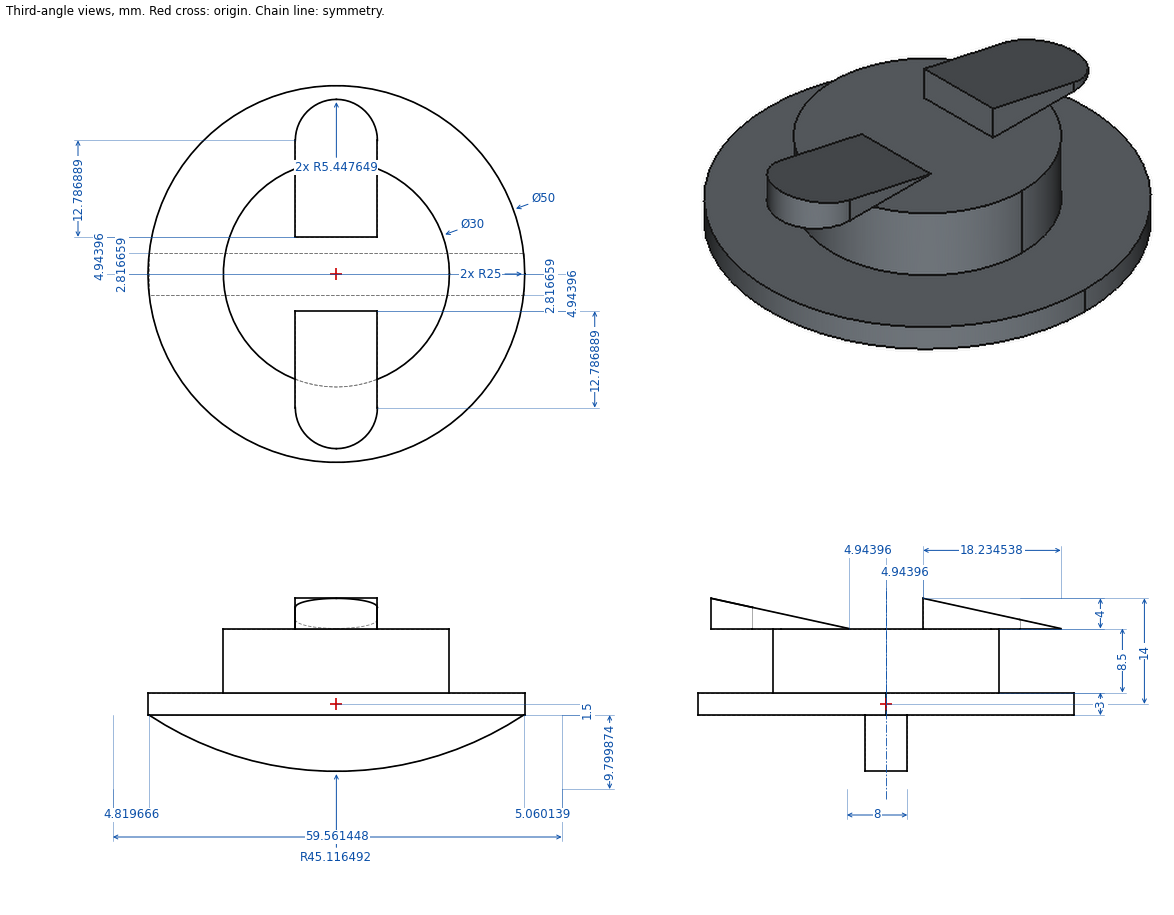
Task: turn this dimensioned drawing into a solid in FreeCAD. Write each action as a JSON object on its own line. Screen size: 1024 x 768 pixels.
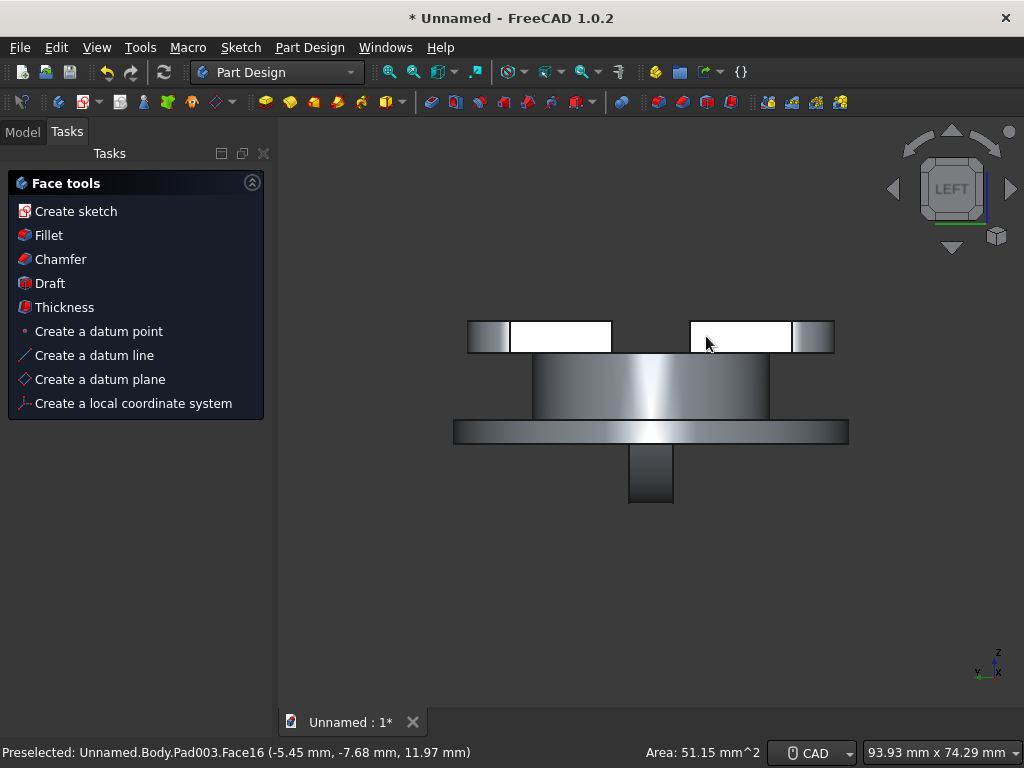
{"action": "left_click", "coordinate": [84, 102]}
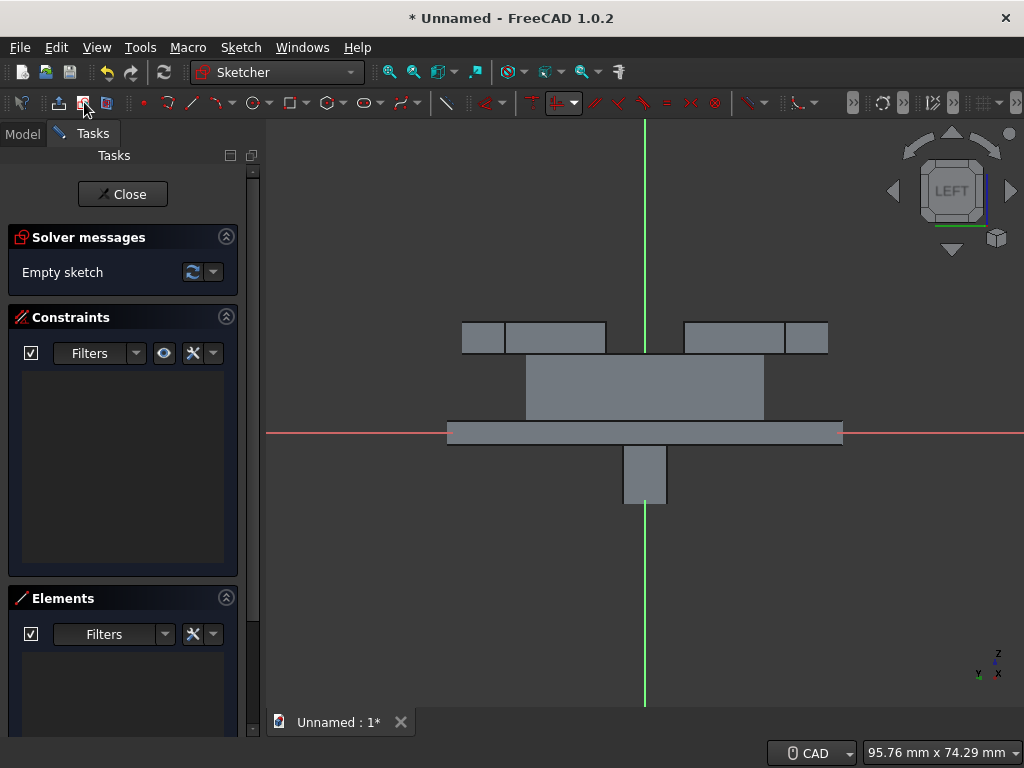
{"action": "left_click", "coordinate": [168, 104]}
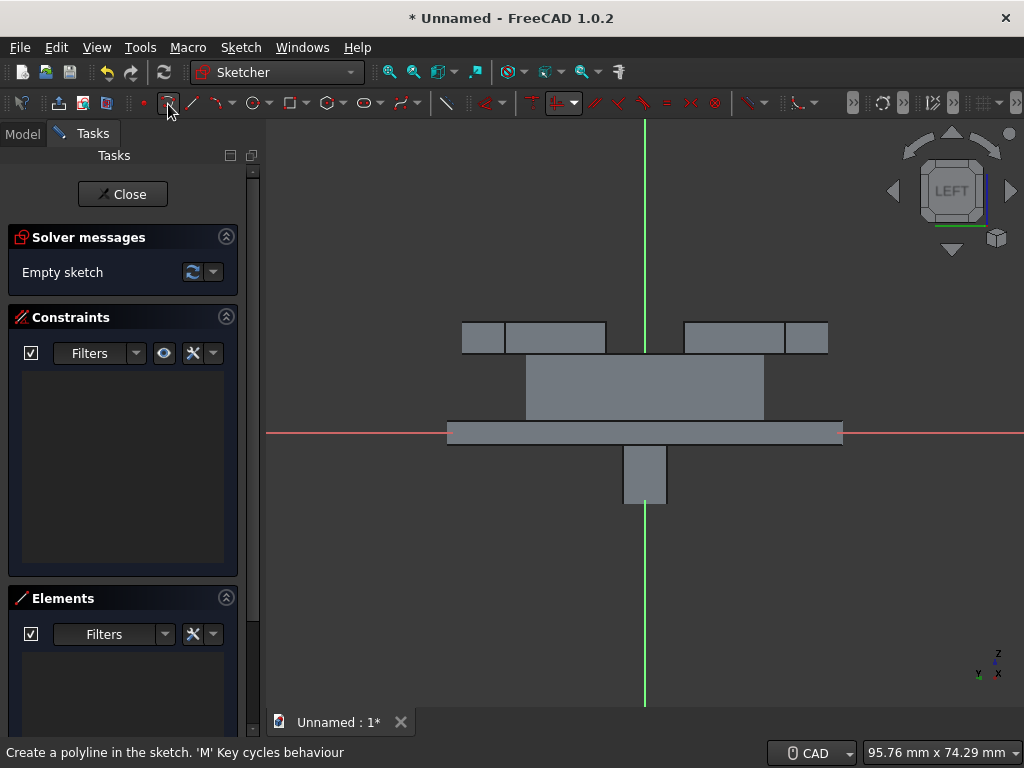
{"action": "left_click", "coordinate": [606, 322]}
{"action": "left_click", "coordinate": [462, 322]}
{"action": "left_click", "coordinate": [462, 354]}
{"action": "left_click", "coordinate": [606, 323]}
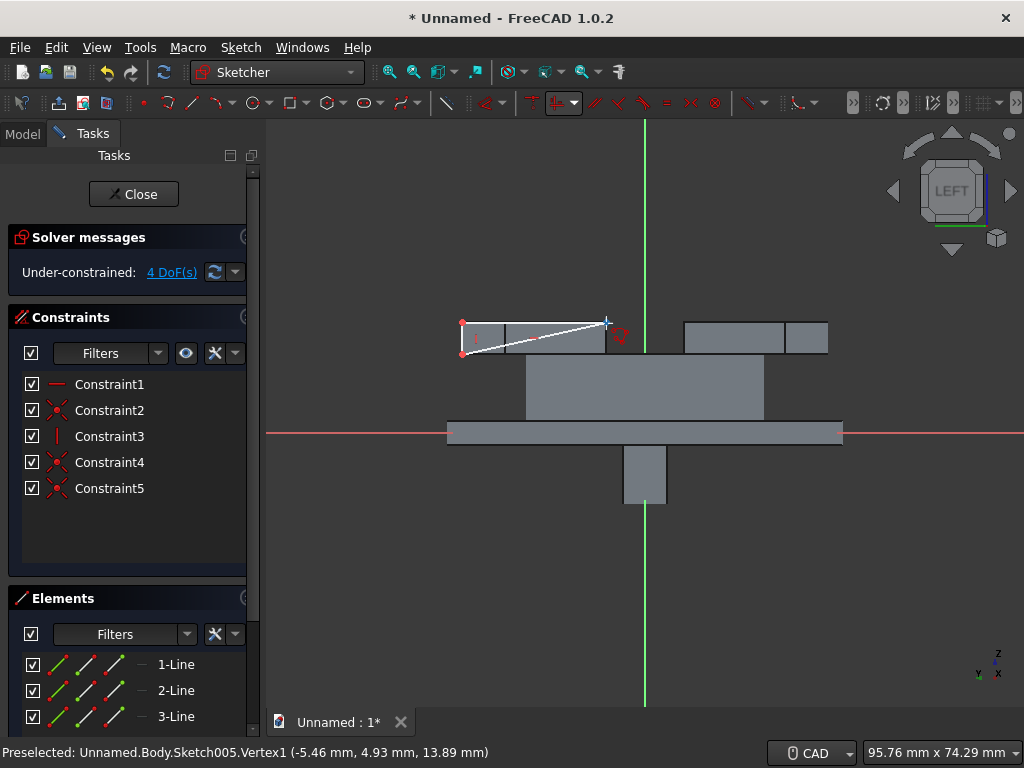
{"action": "left_click", "coordinate": [684, 354]}
{"action": "left_click", "coordinate": [828, 322]}
{"action": "left_click", "coordinate": [684, 322]}
{"action": "left_click", "coordinate": [684, 355]}
{"action": "key", "text": "Escape"}
{"action": "key", "text": "Escape"}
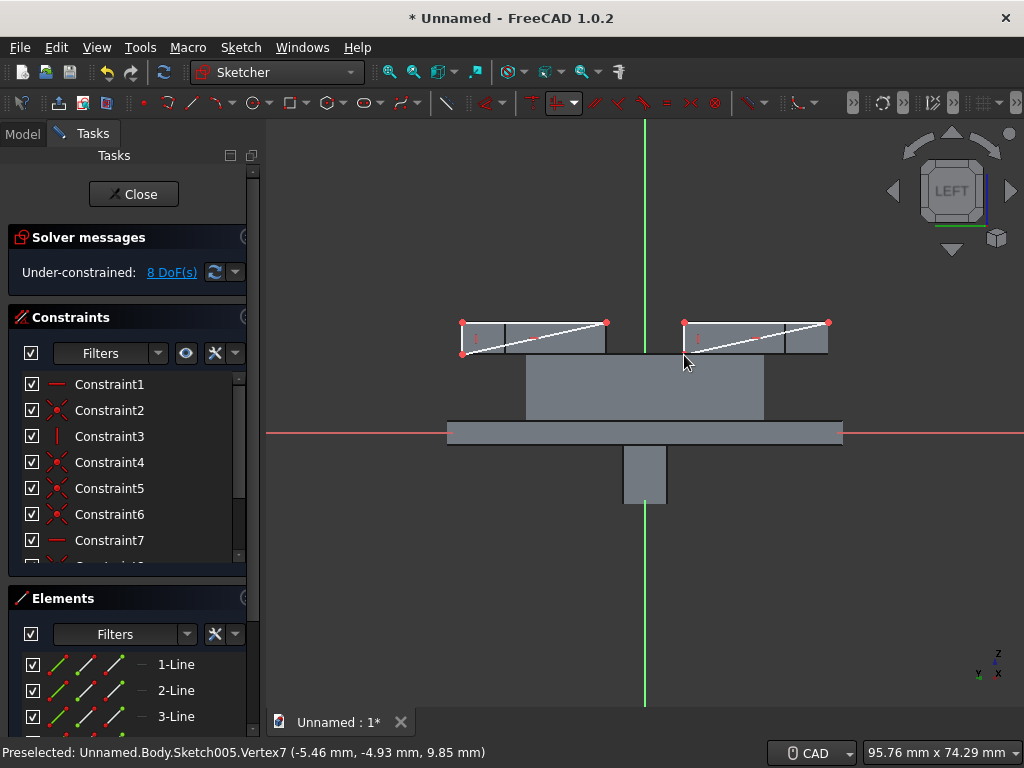
{"action": "left_click", "coordinate": [462, 323]}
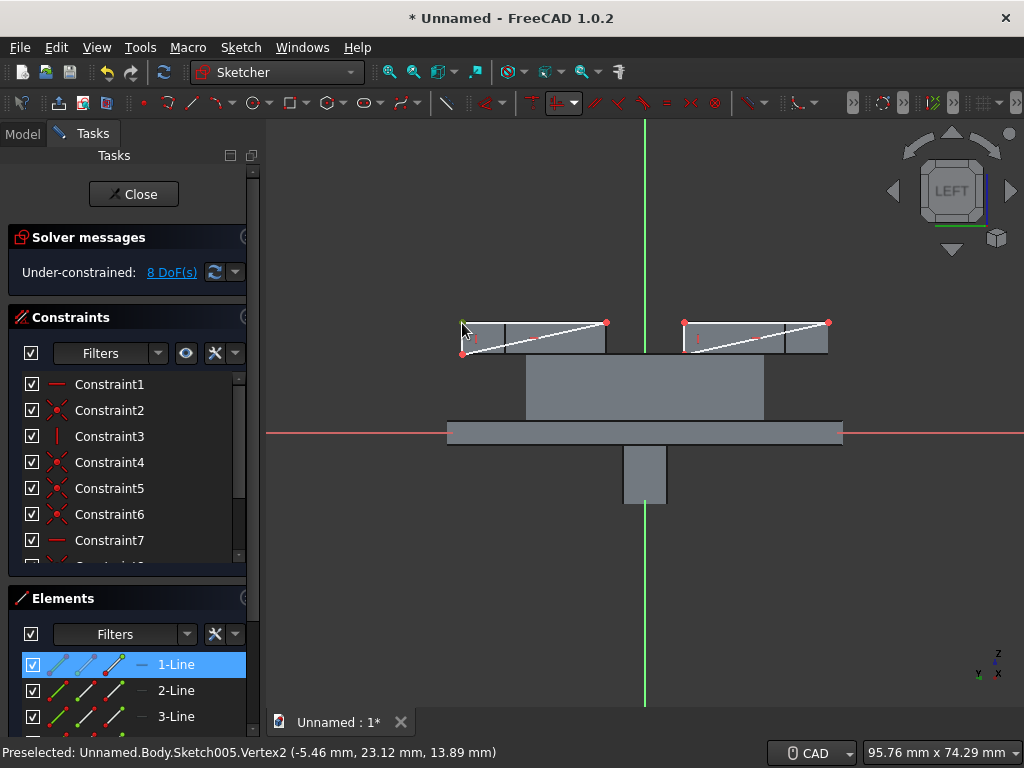
{"action": "left_click", "coordinate": [828, 323]}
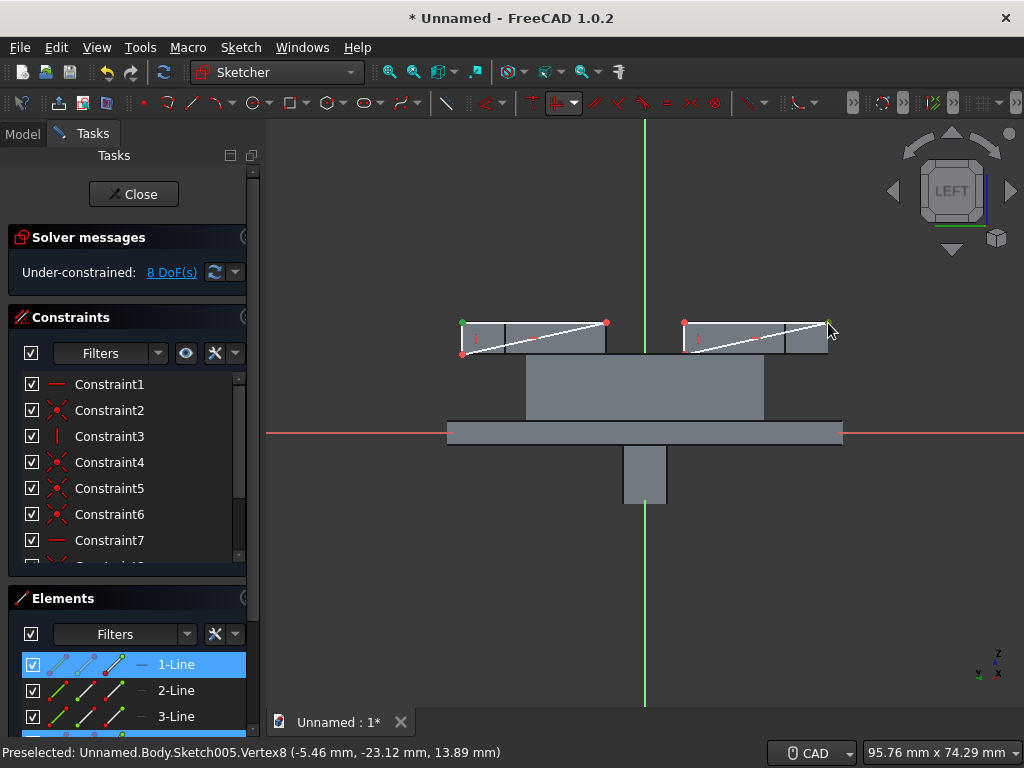
{"action": "left_click", "coordinate": [645, 641]}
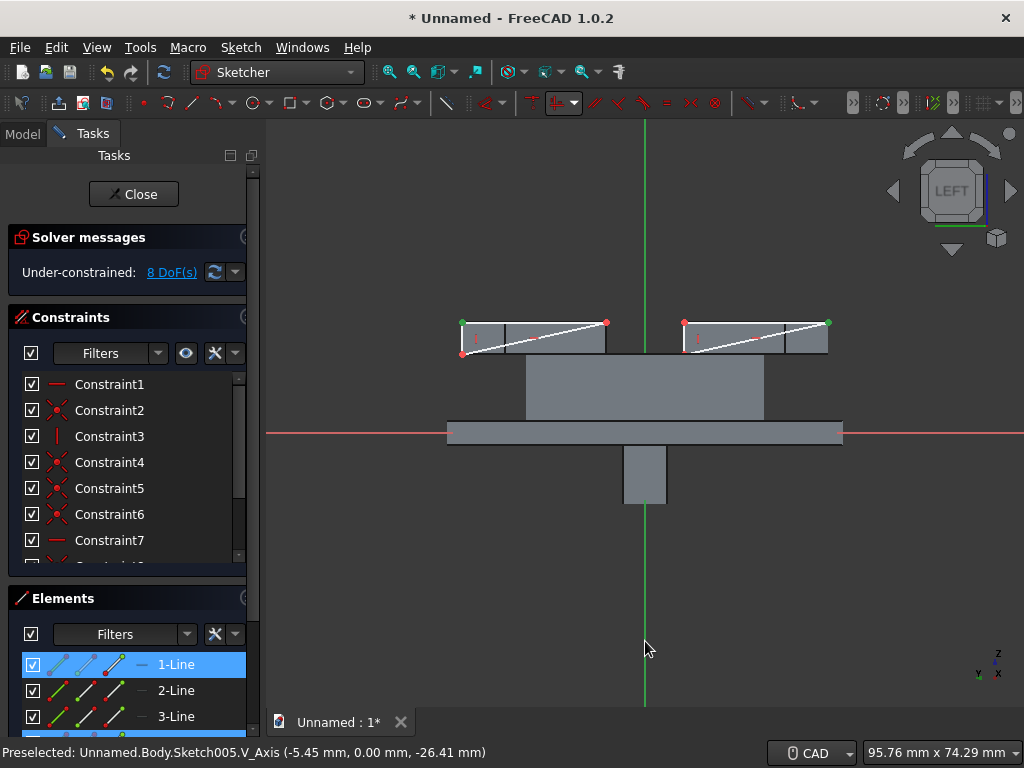
{"action": "left_click", "coordinate": [692, 104]}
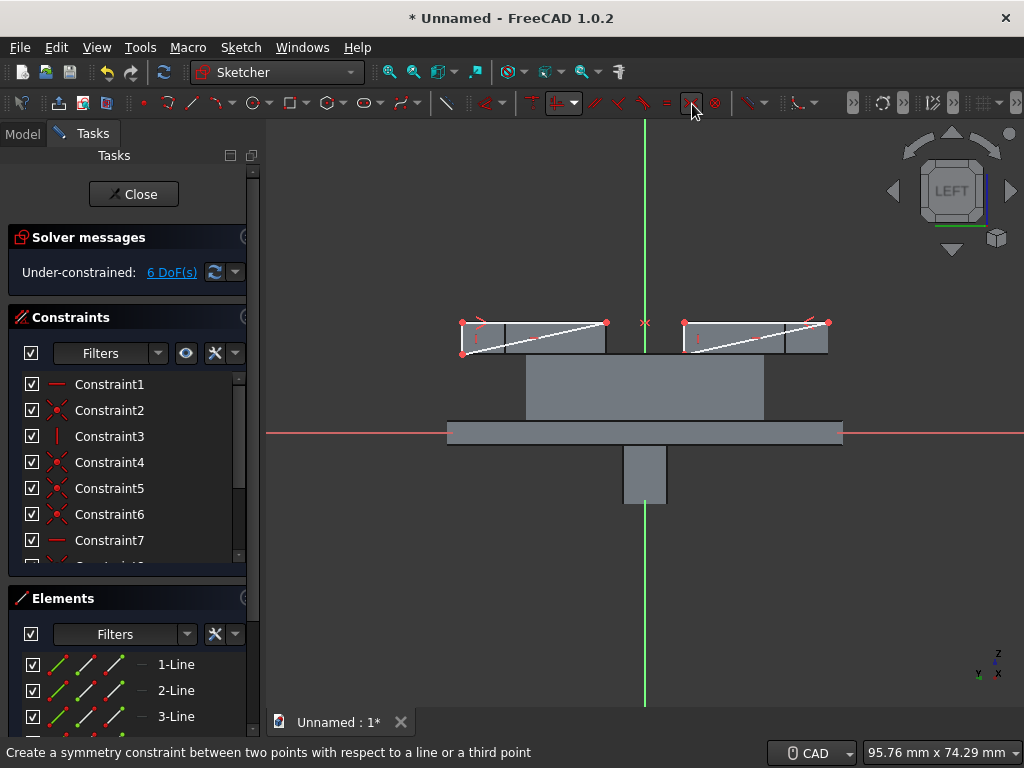
{"action": "left_click", "coordinate": [486, 104]}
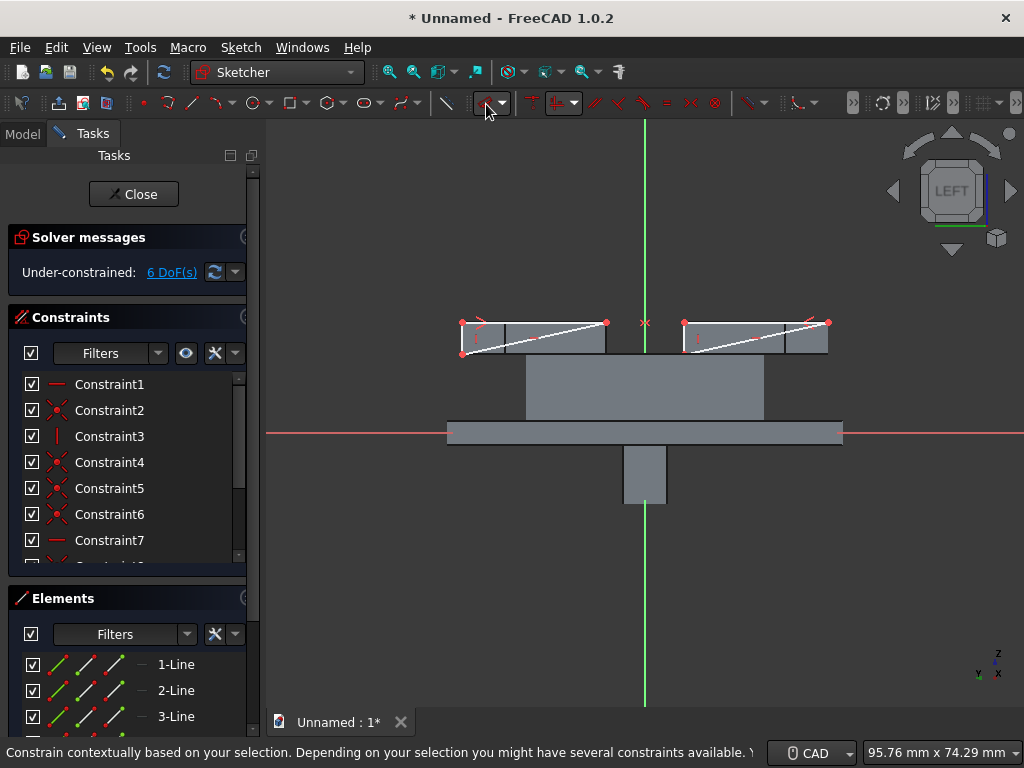
{"action": "scroll", "coordinate": [462, 333], "scroll_direction": "up", "scroll_amount": 2}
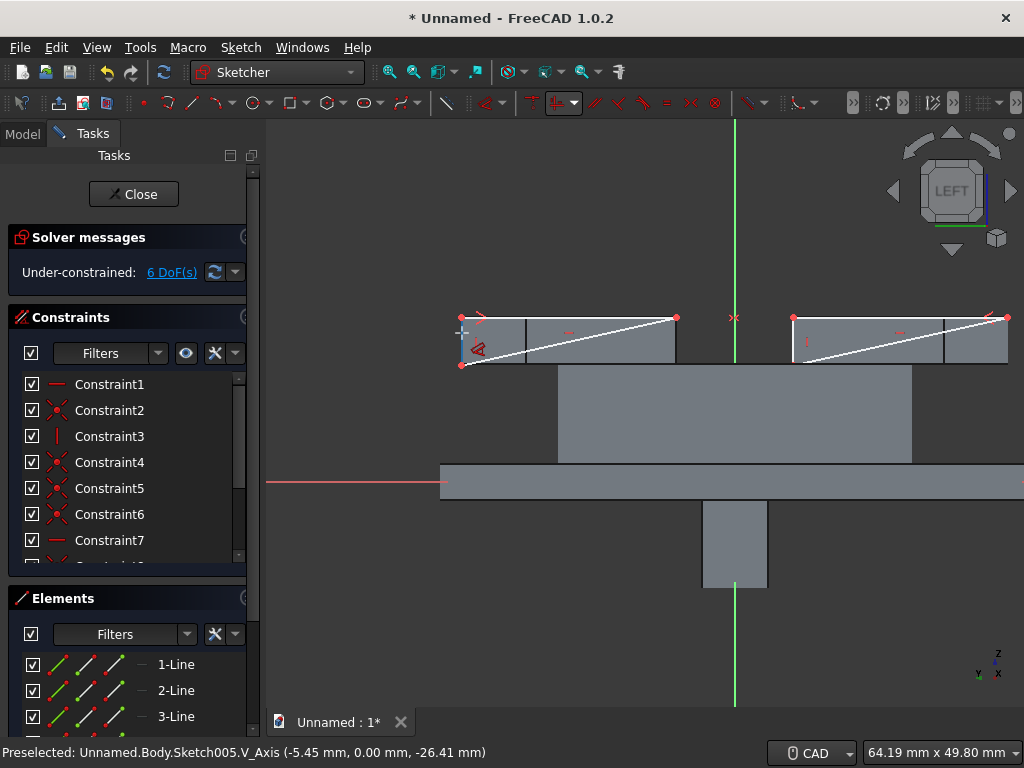
{"action": "left_click", "coordinate": [462, 332]}
{"action": "left_click", "coordinate": [428, 342]}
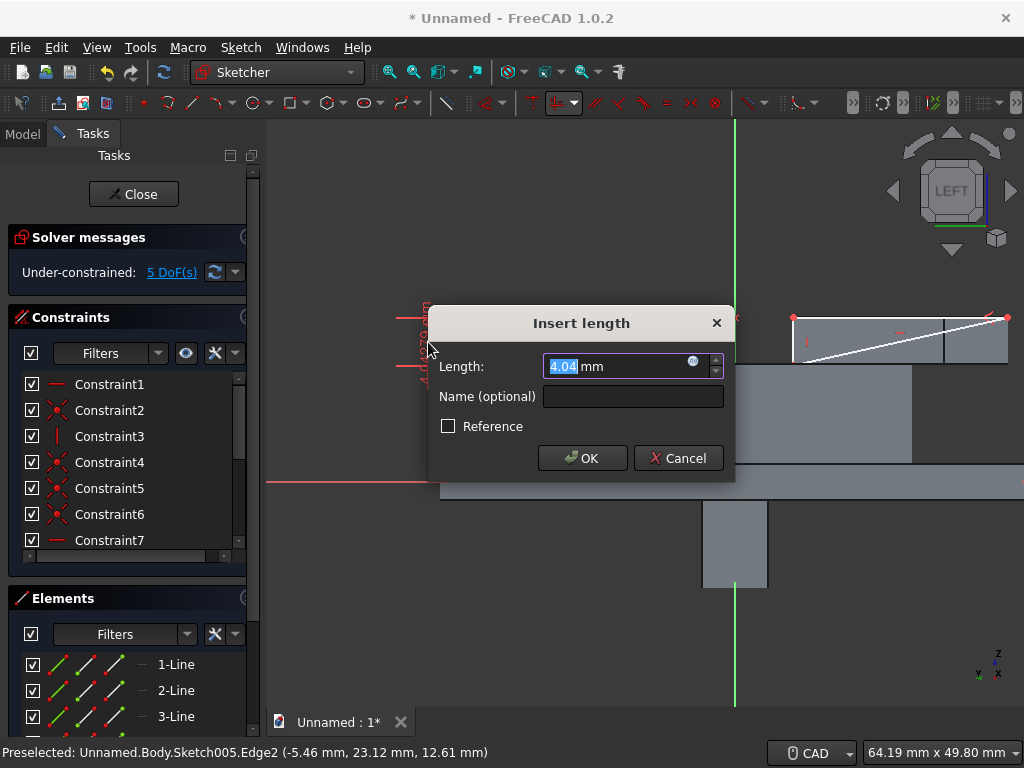
{"action": "type", "text": "4"}
{"action": "key", "text": "Return"}